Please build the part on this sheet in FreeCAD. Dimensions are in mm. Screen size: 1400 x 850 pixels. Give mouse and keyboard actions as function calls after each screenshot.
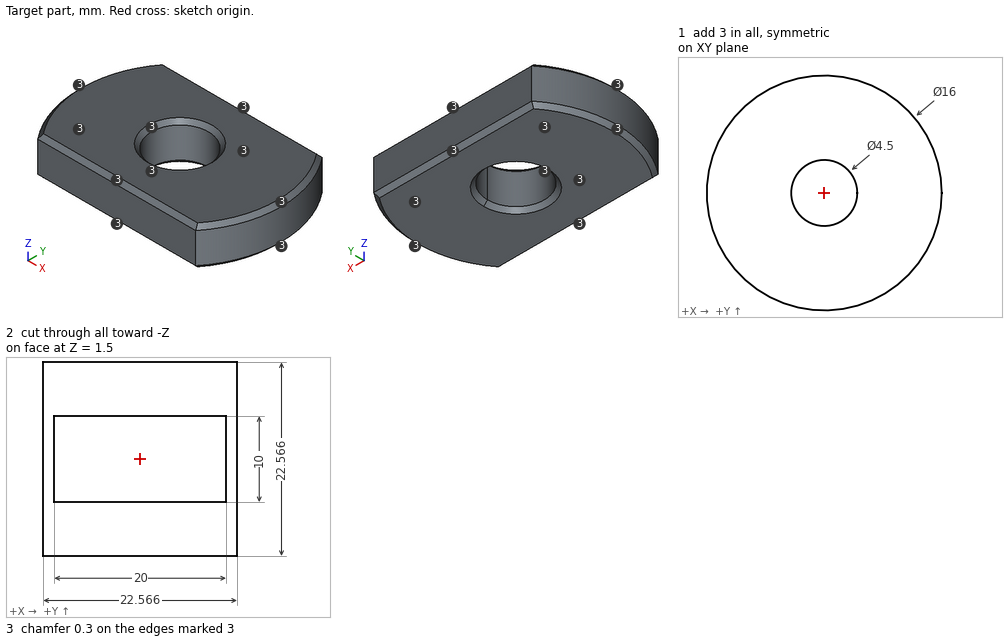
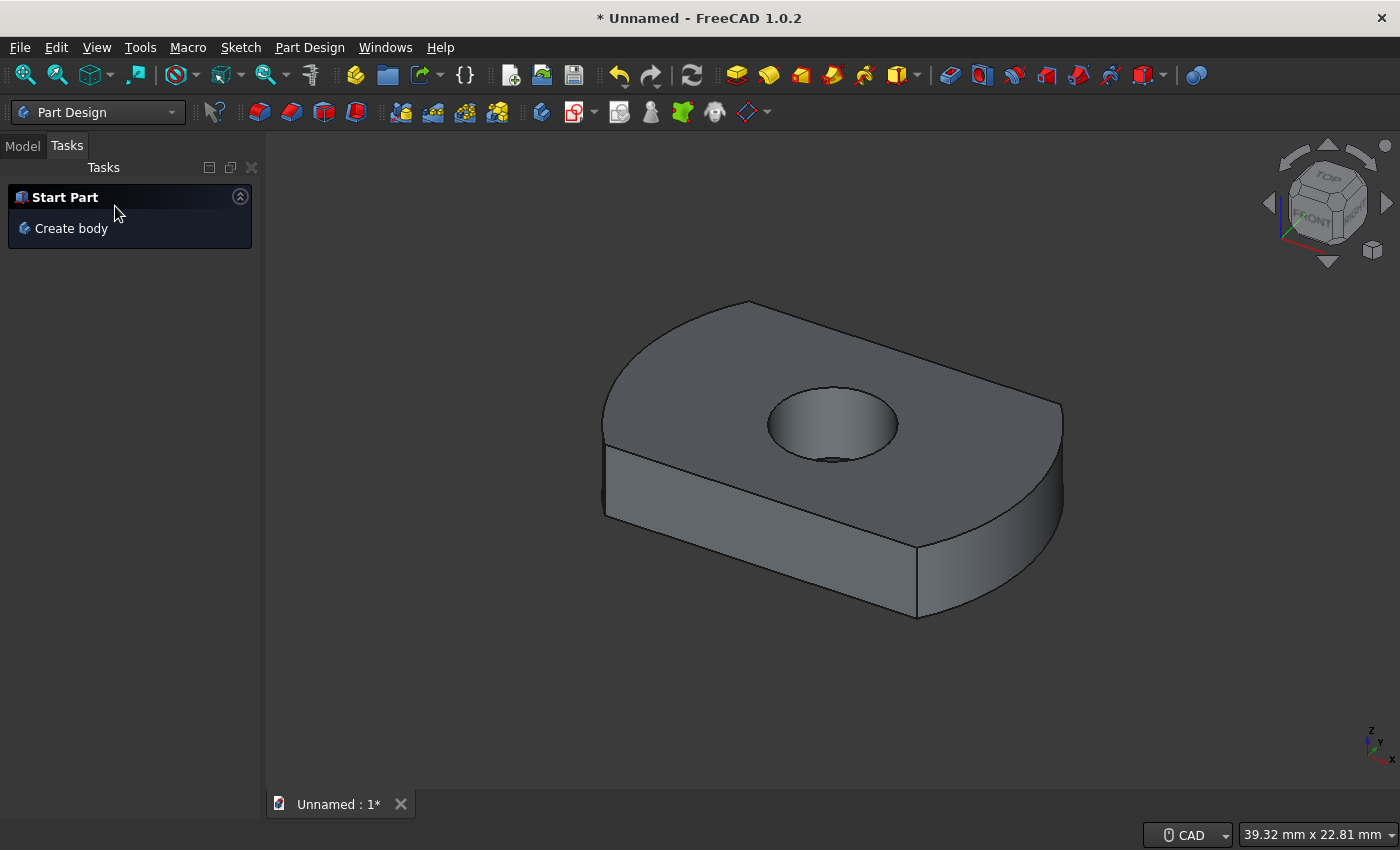
click(983, 524)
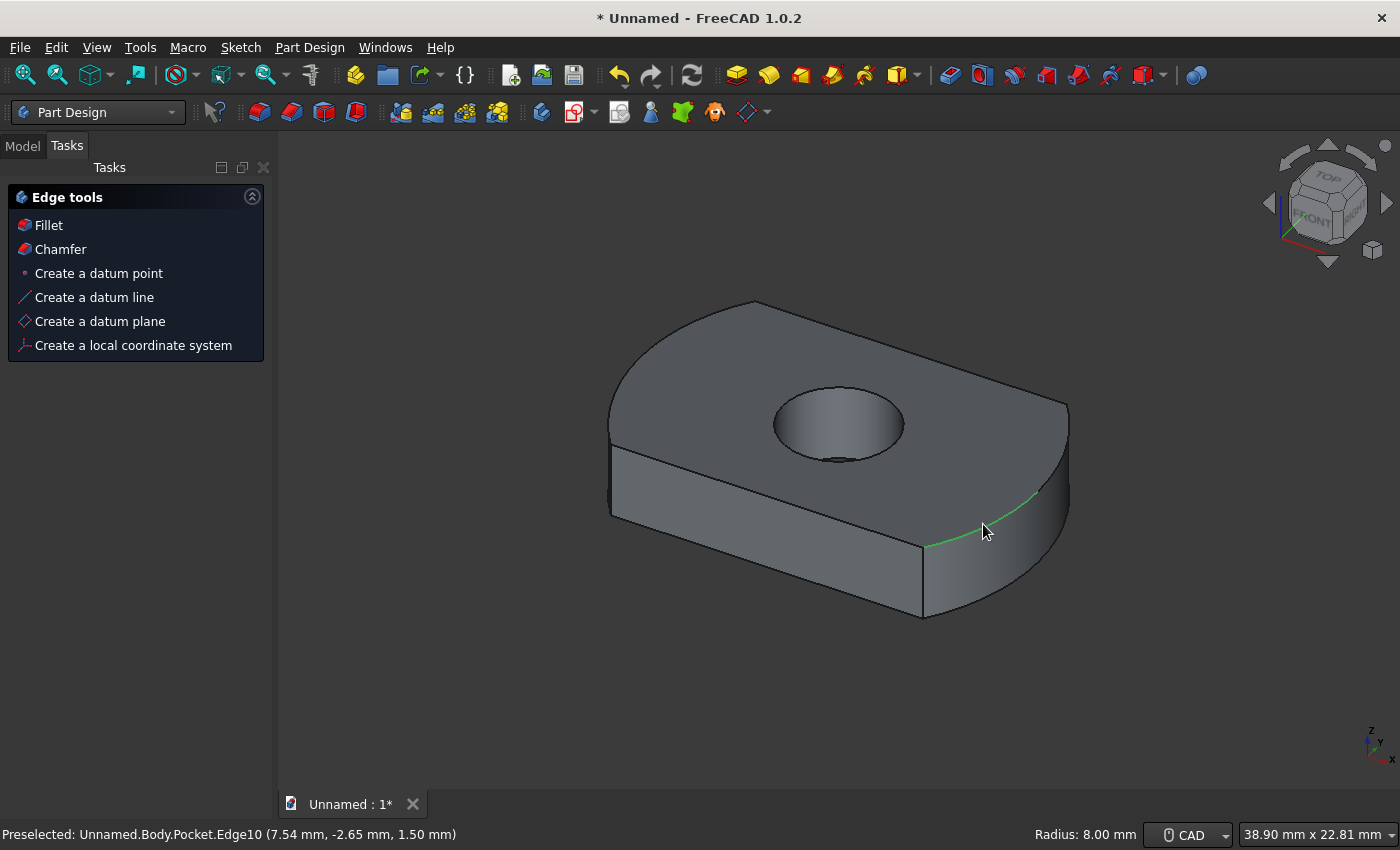
click(1001, 589, ctrl)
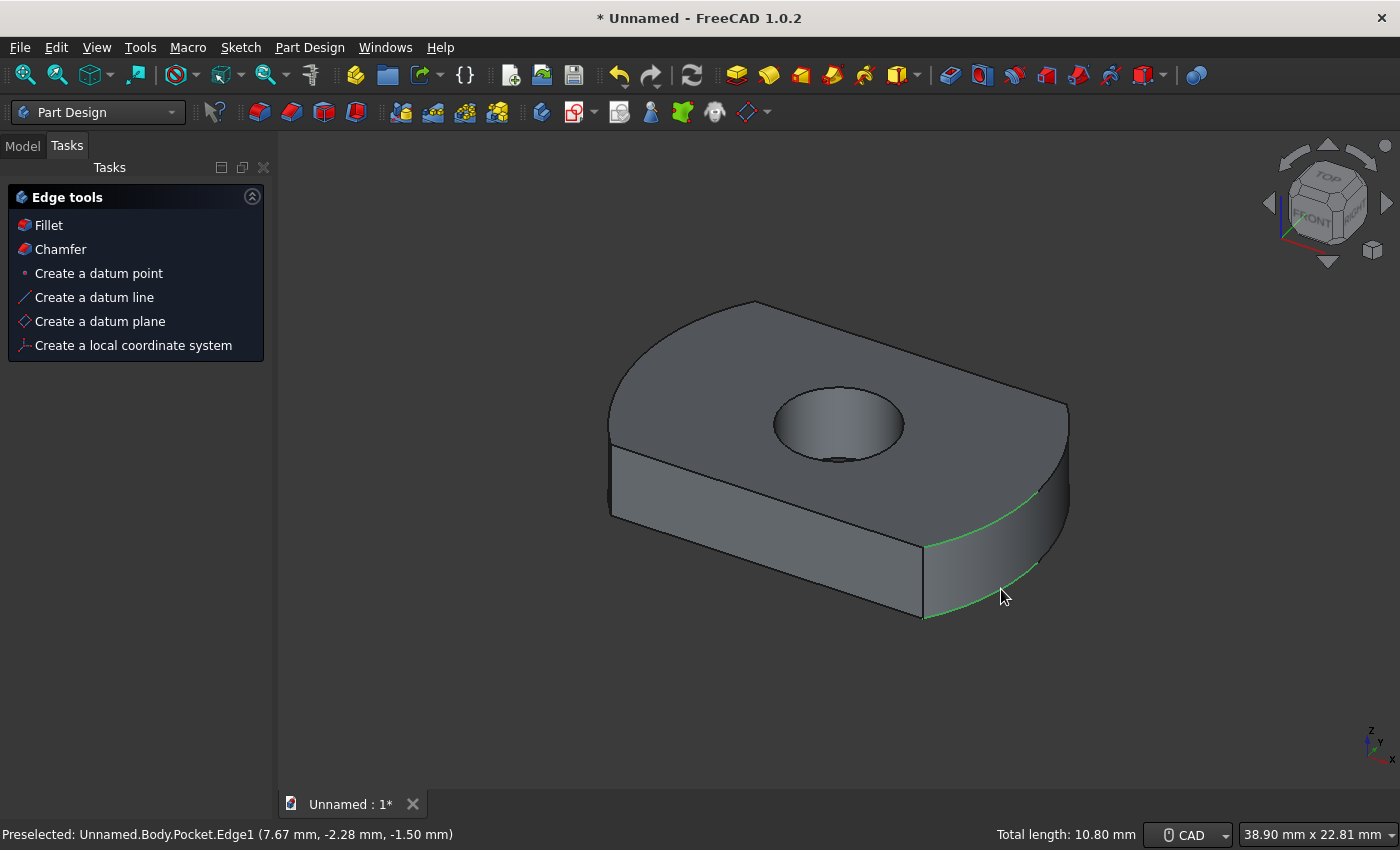
click(767, 495, ctrl)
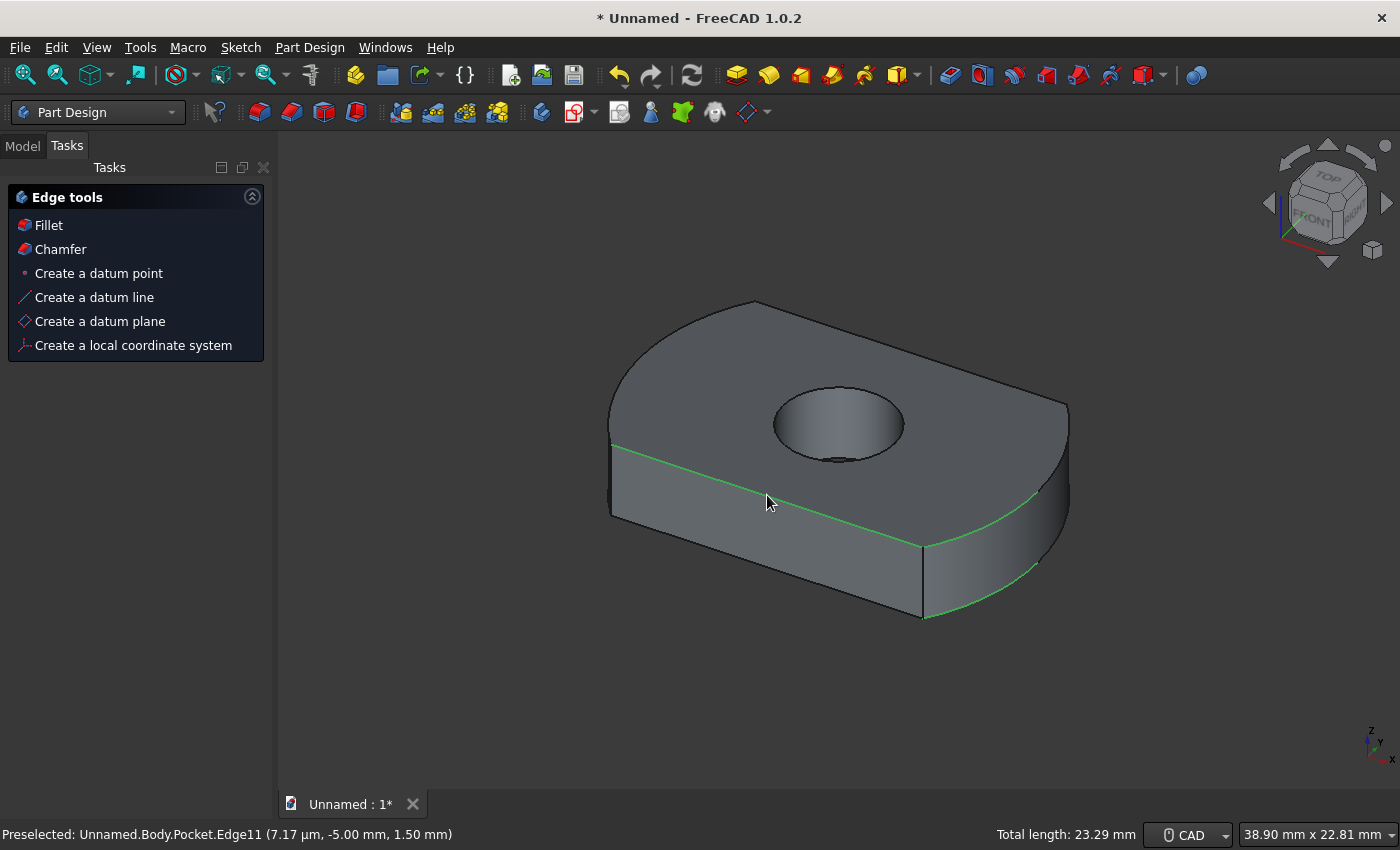
click(783, 405, ctrl)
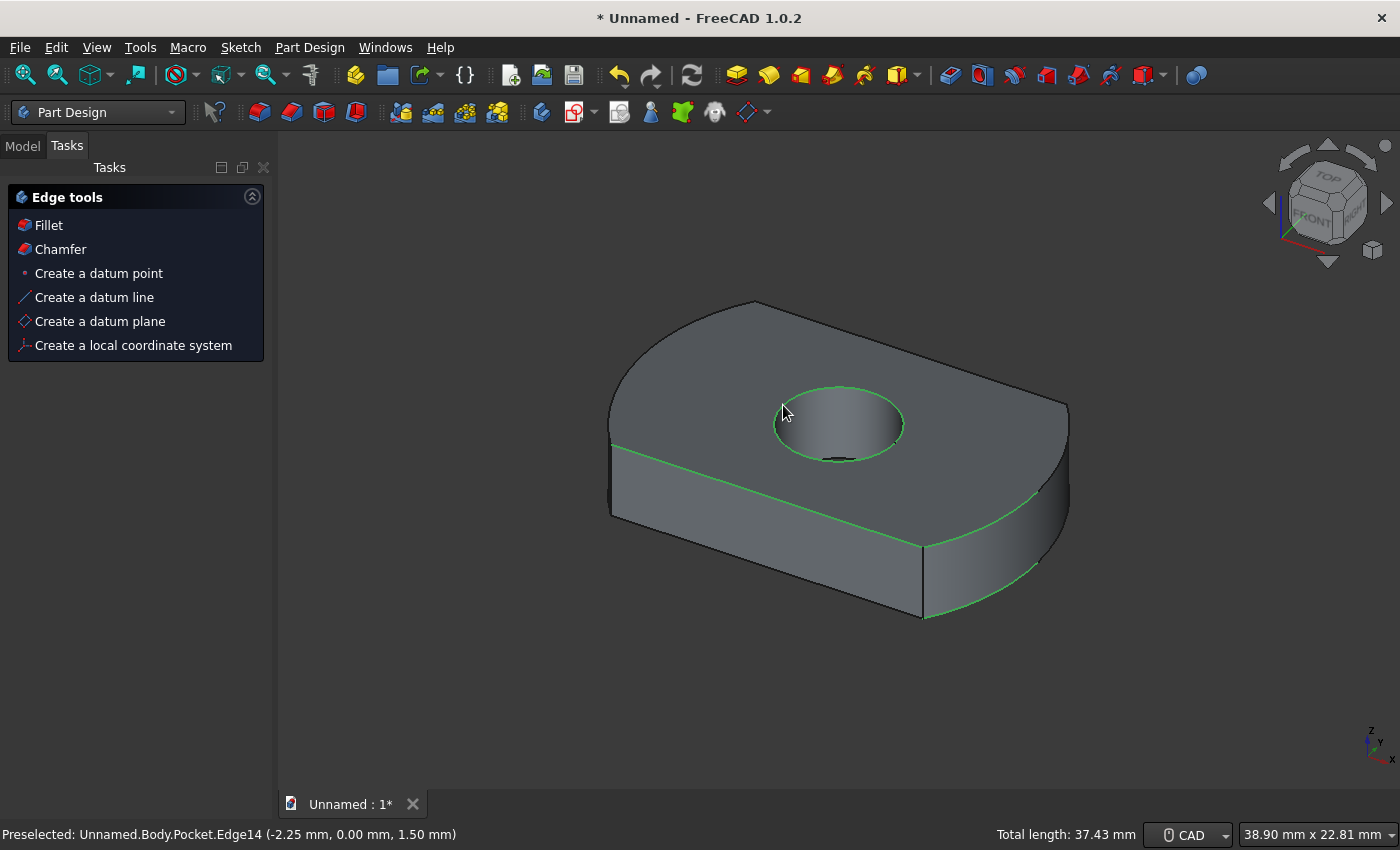
click(615, 390, ctrl)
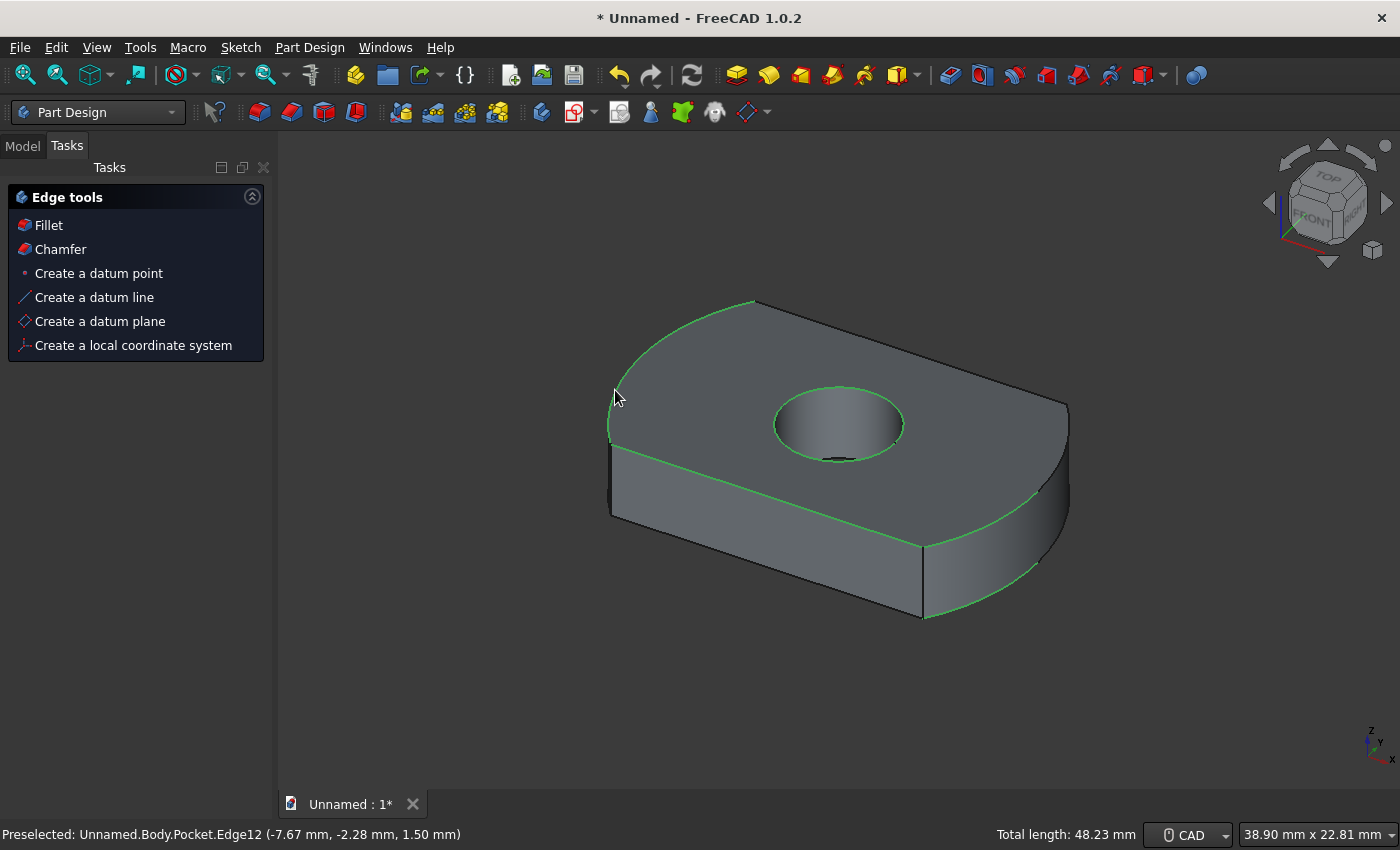
key(0)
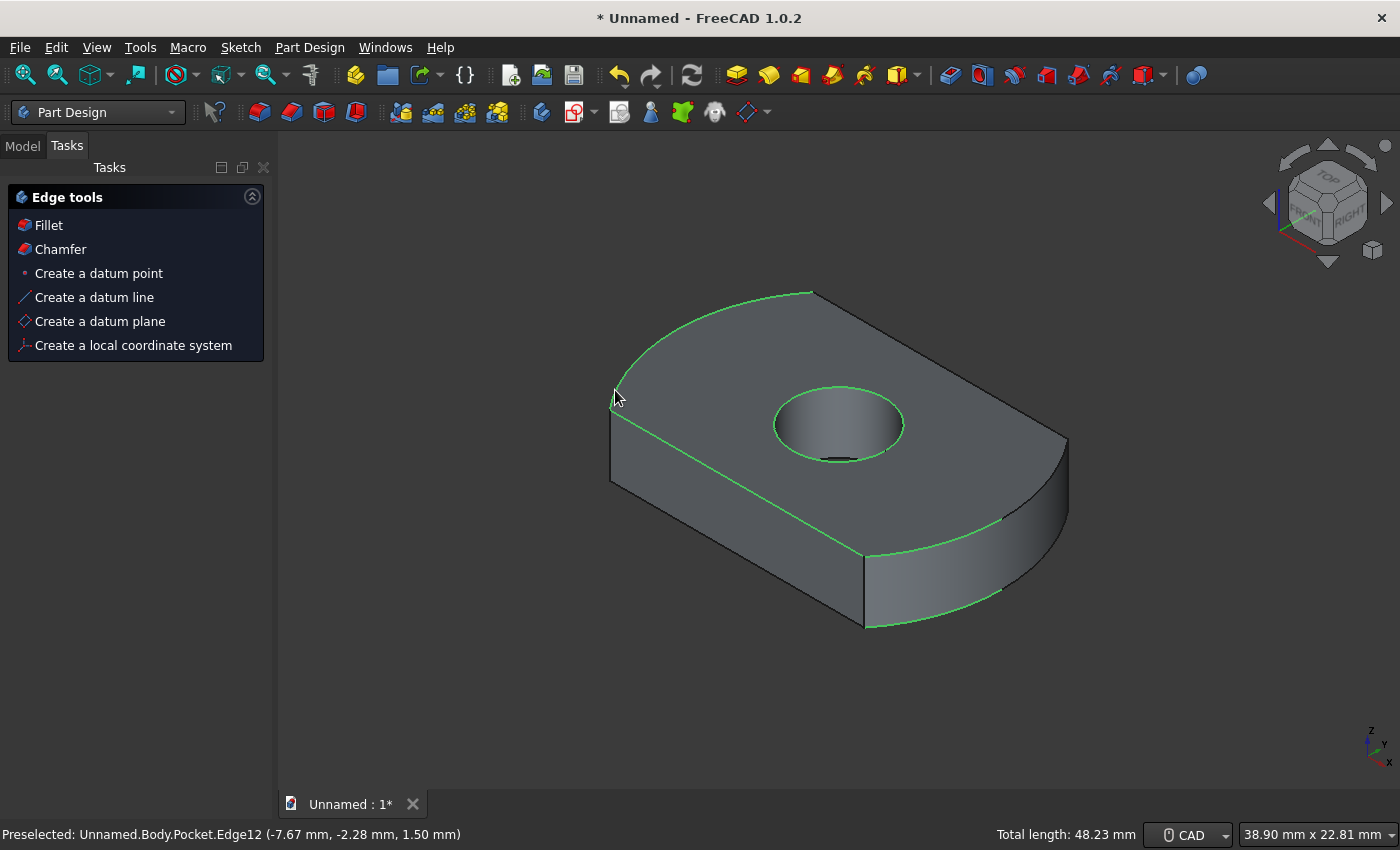
key(2)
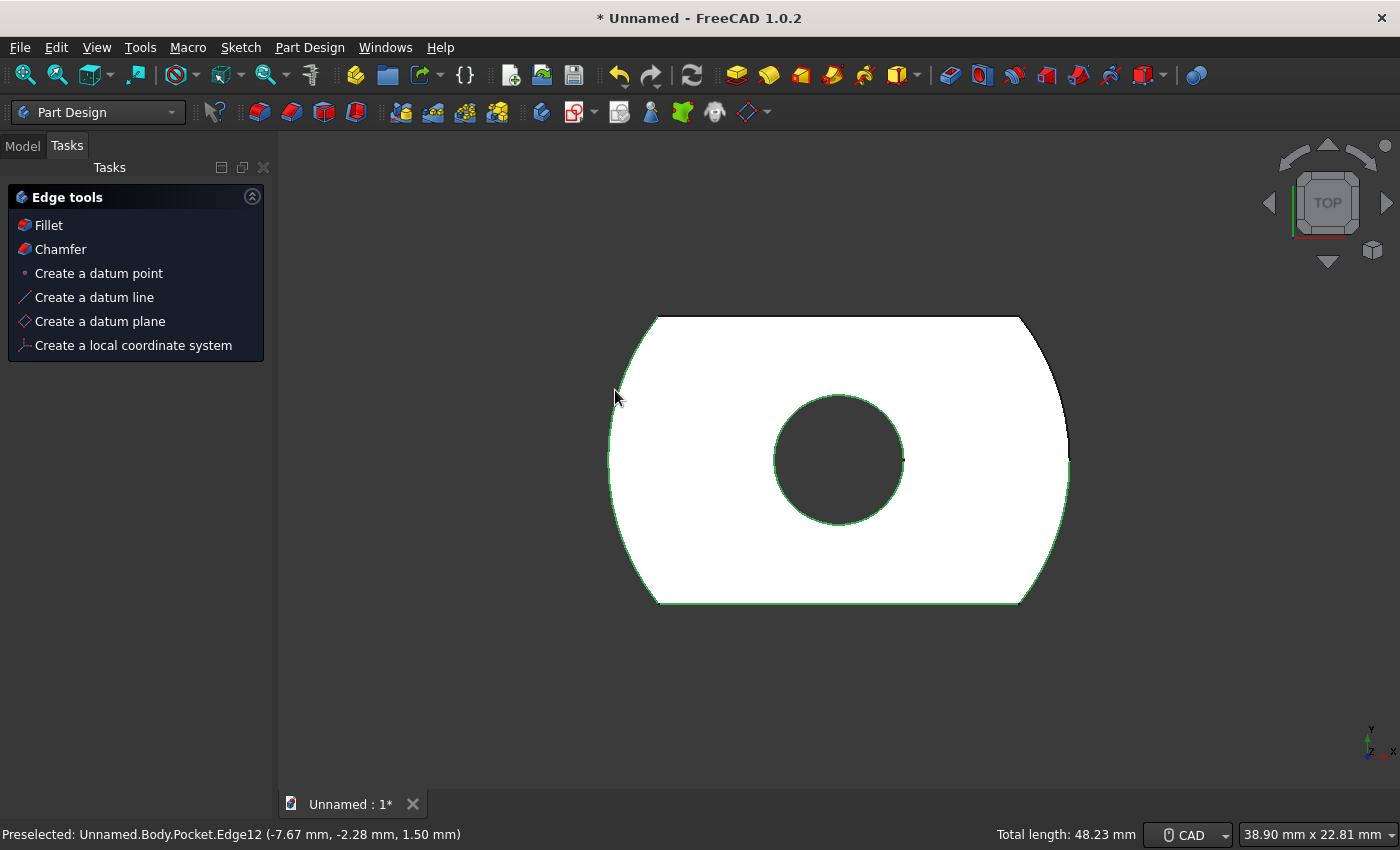
key(v)
key(f)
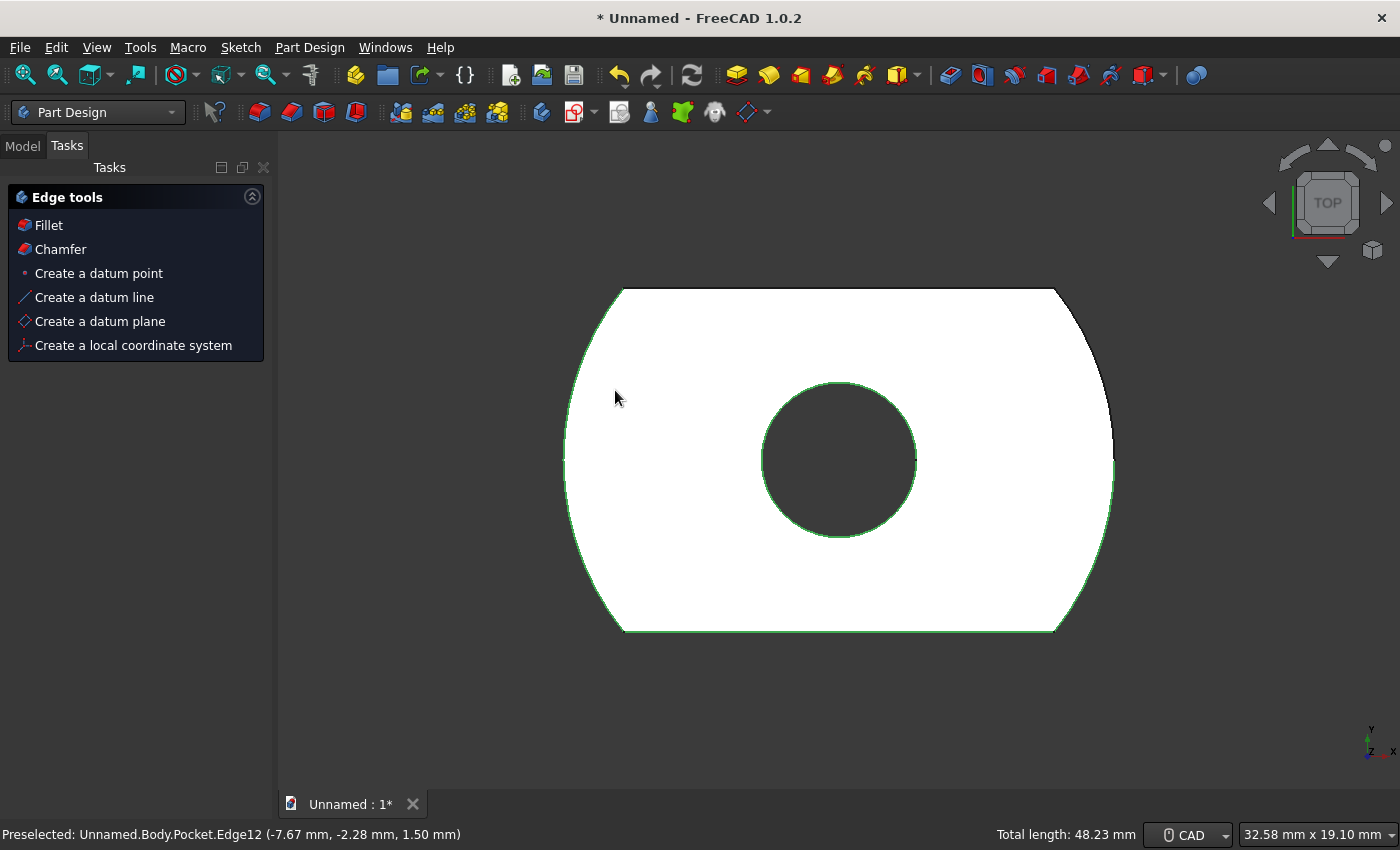
click(839, 287, ctrl)